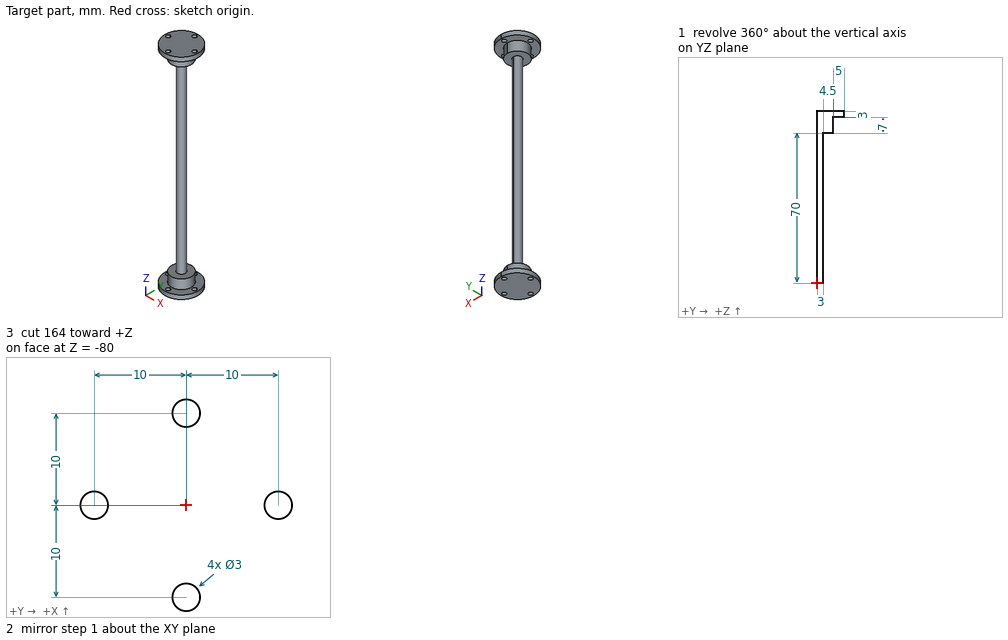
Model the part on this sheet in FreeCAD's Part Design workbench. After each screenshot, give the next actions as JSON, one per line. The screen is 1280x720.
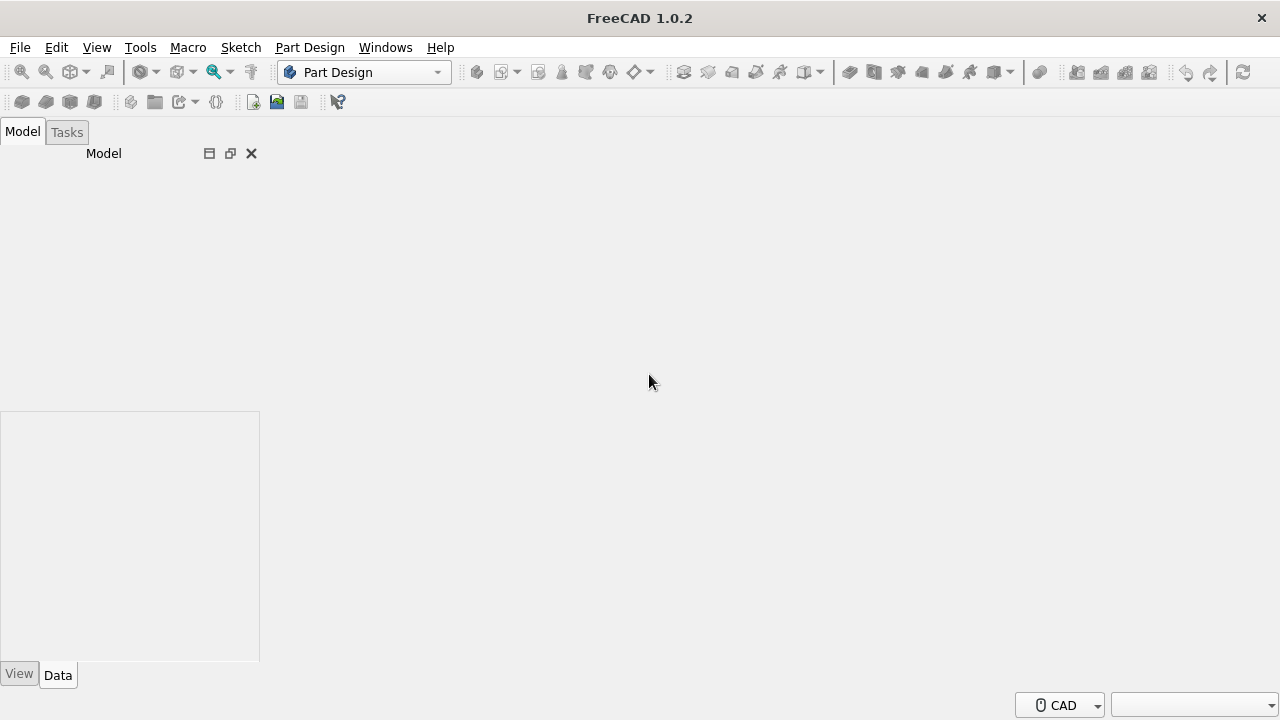
{"action": "left_click", "coordinate": [254, 102]}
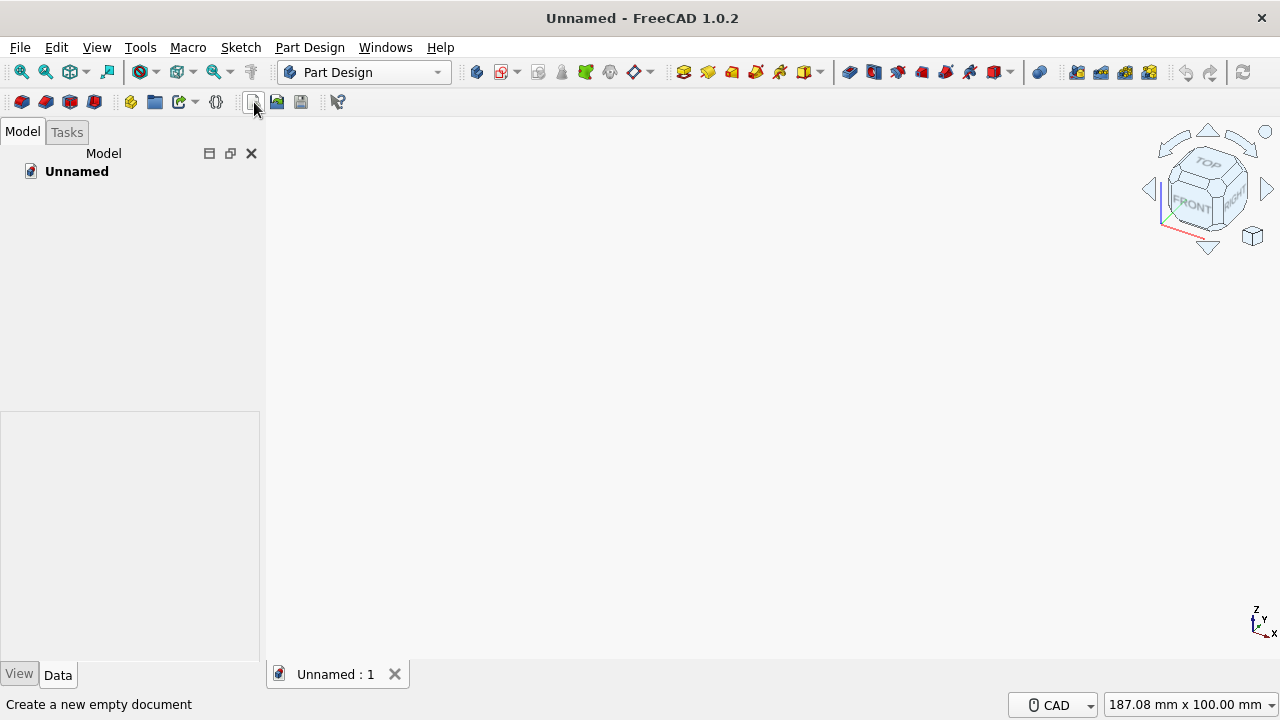
{"action": "left_click", "coordinate": [502, 72]}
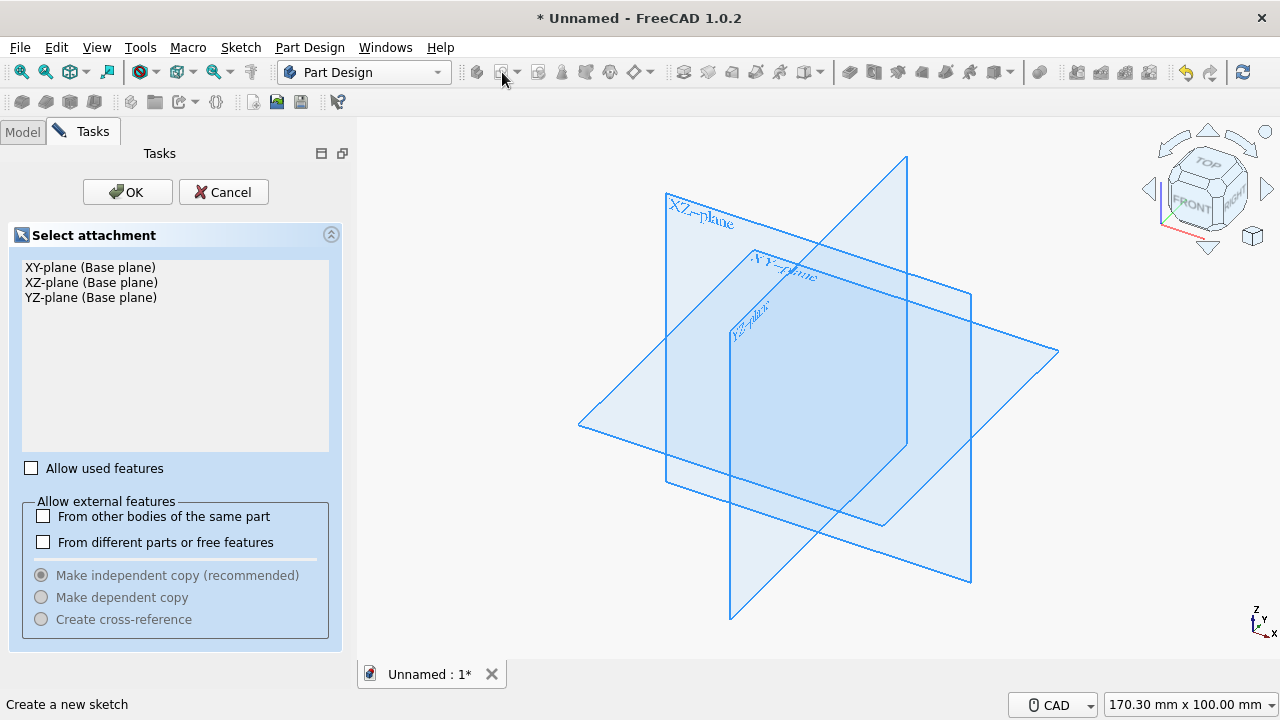
{"action": "left_click", "coordinate": [82, 298]}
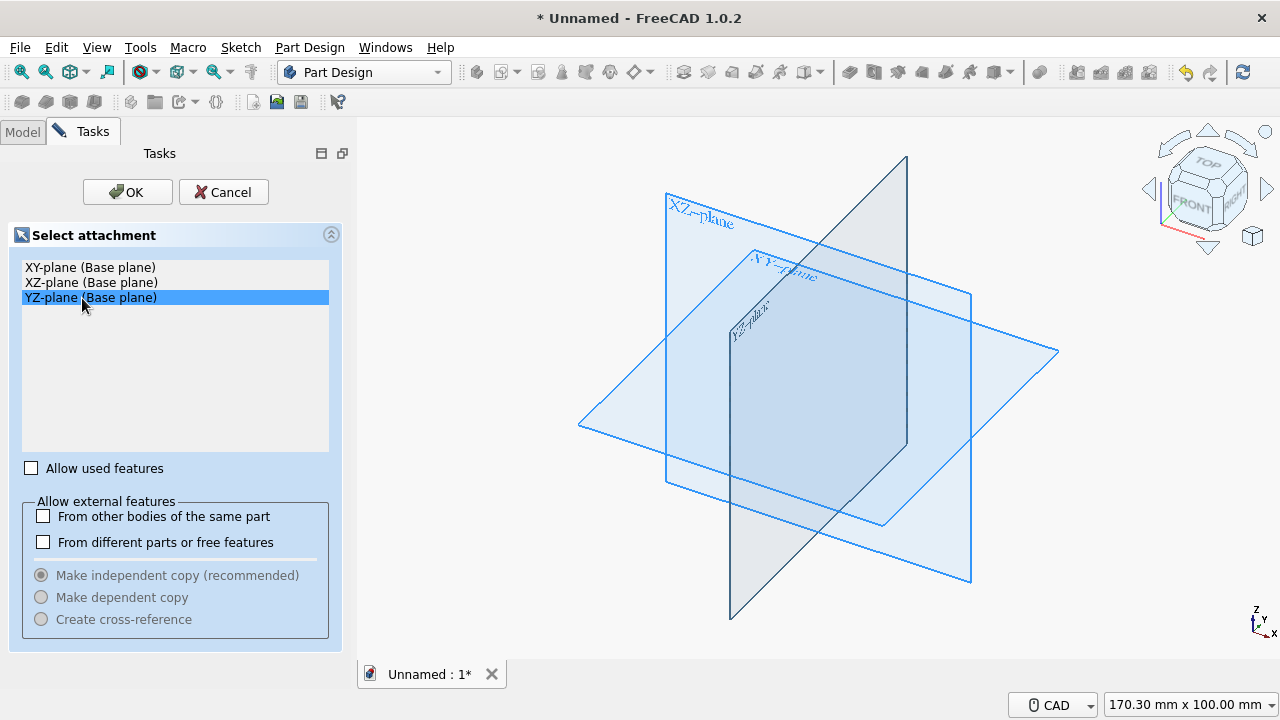
{"action": "left_click", "coordinate": [128, 192]}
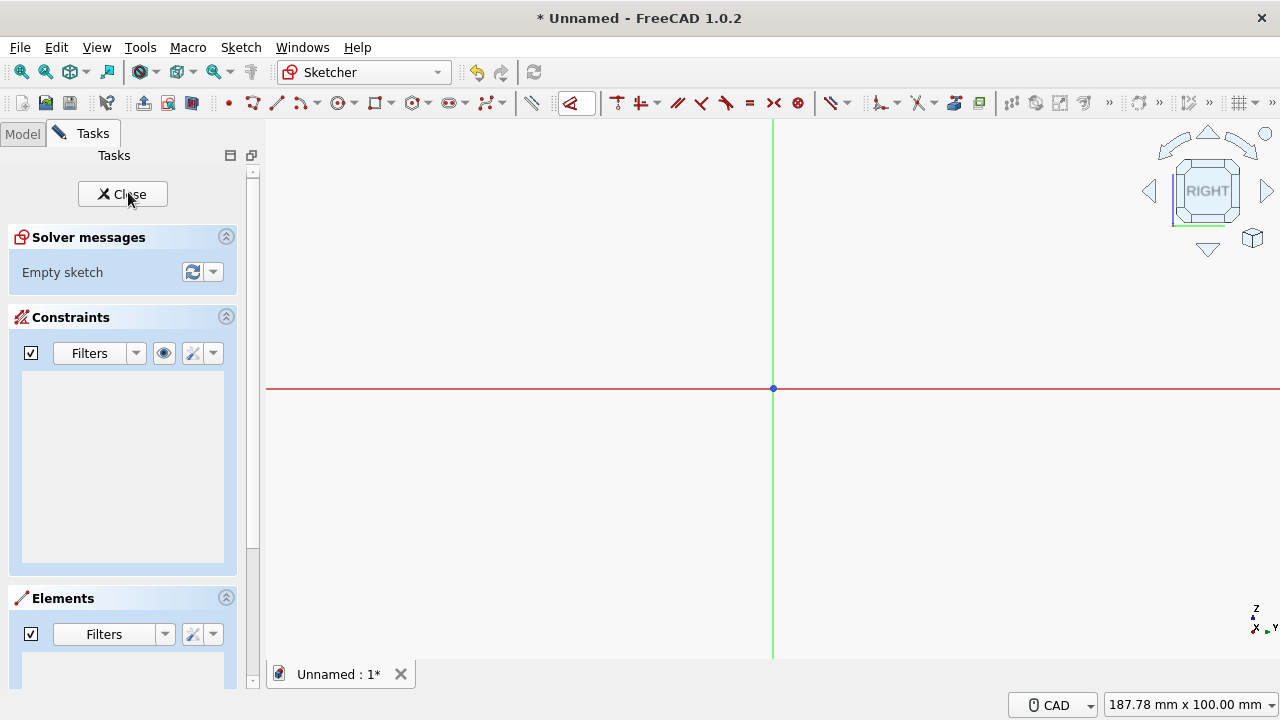
{"action": "scroll", "coordinate": [497, 631], "scroll_direction": "down", "scroll_amount": 2}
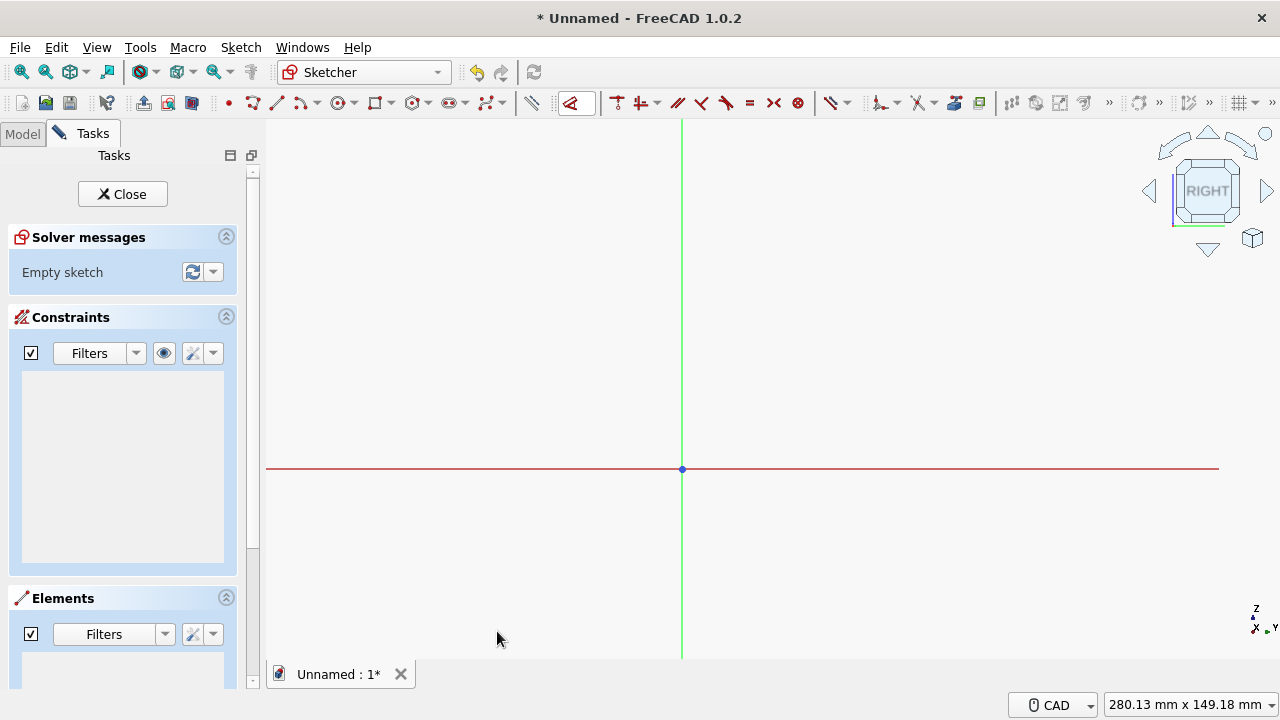
{"action": "left_click", "coordinate": [254, 104]}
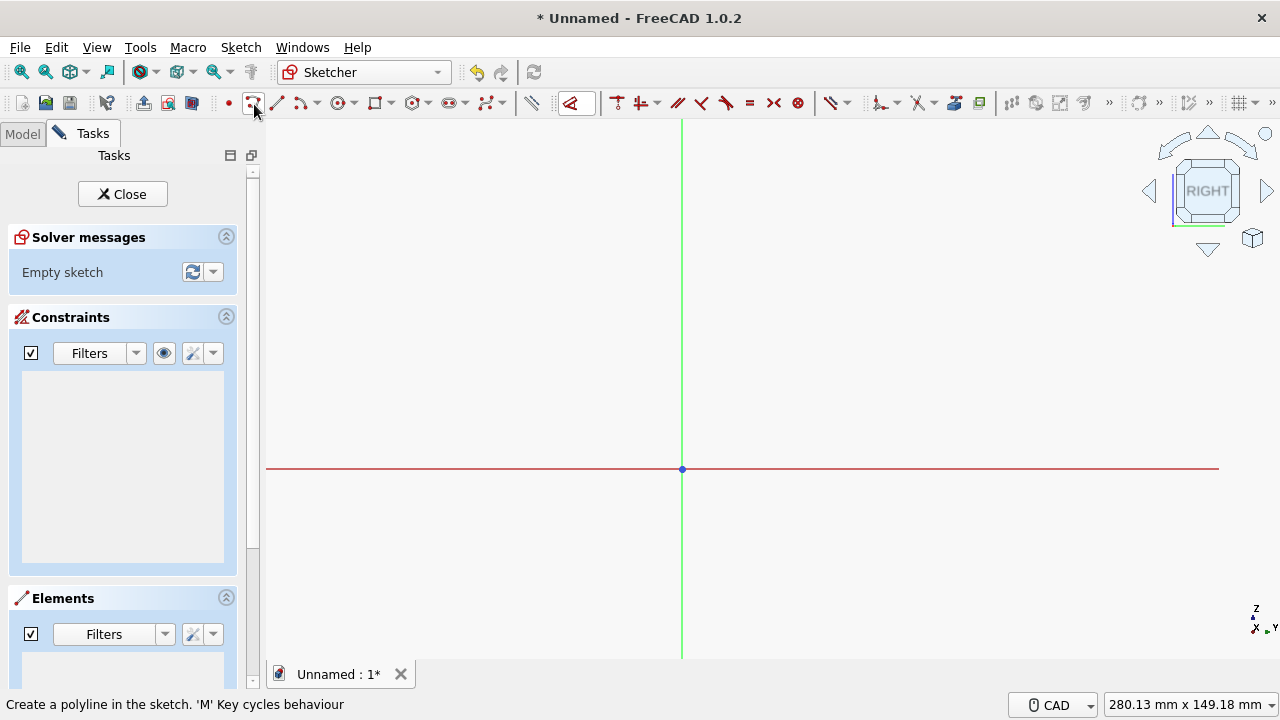
{"action": "left_click", "coordinate": [682, 469]}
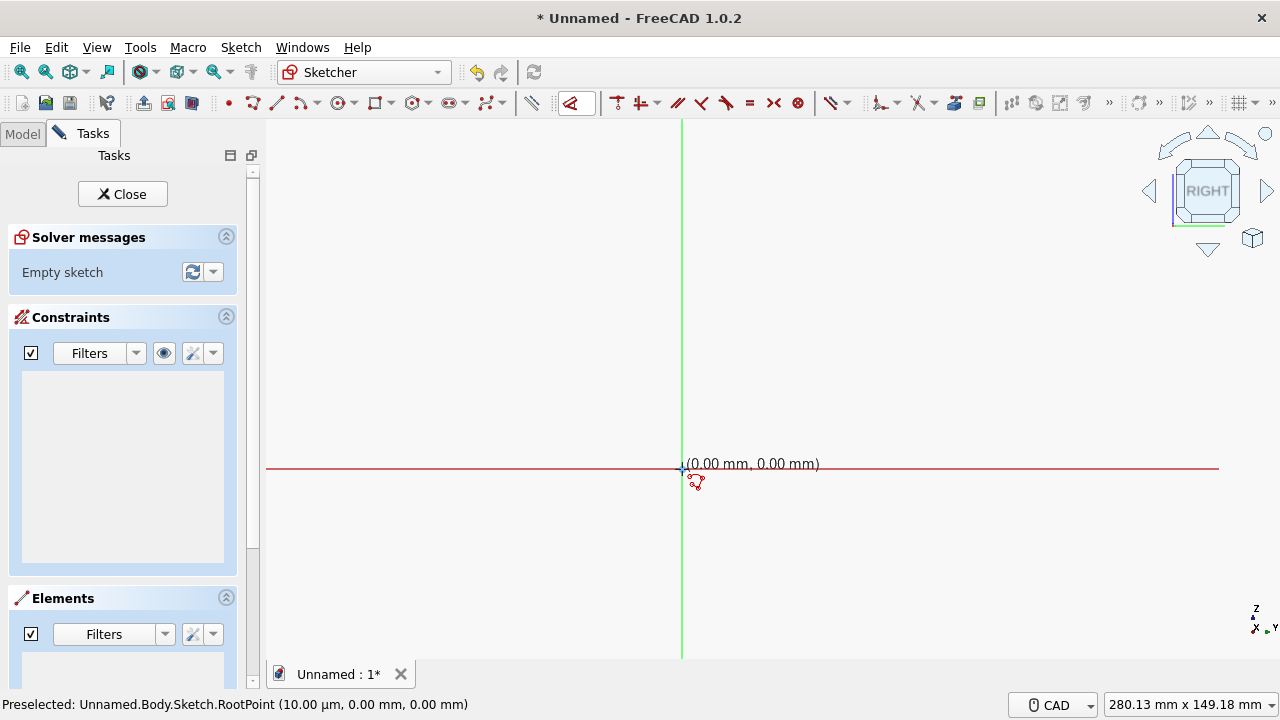
{"action": "scroll", "coordinate": [693, 469], "scroll_direction": "up", "scroll_amount": 2}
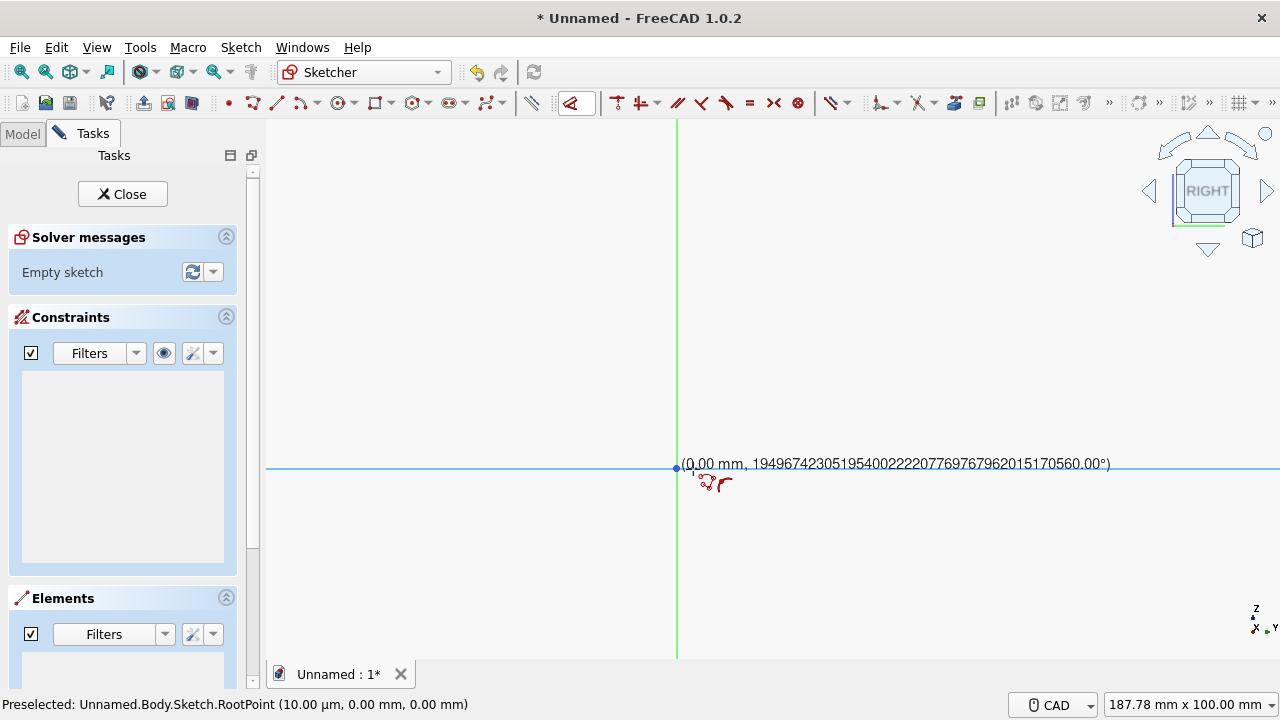
{"action": "left_click", "coordinate": [693, 460]}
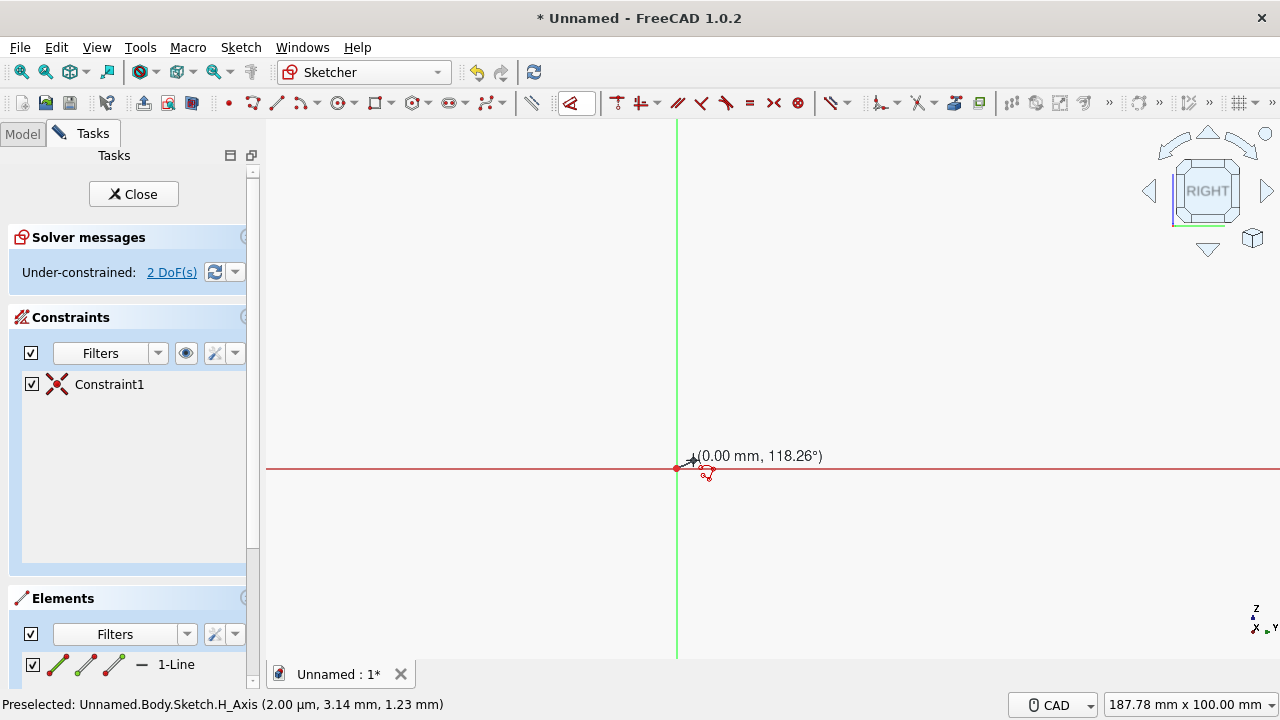
{"action": "scroll", "coordinate": [693, 631], "scroll_direction": "down", "scroll_amount": 2}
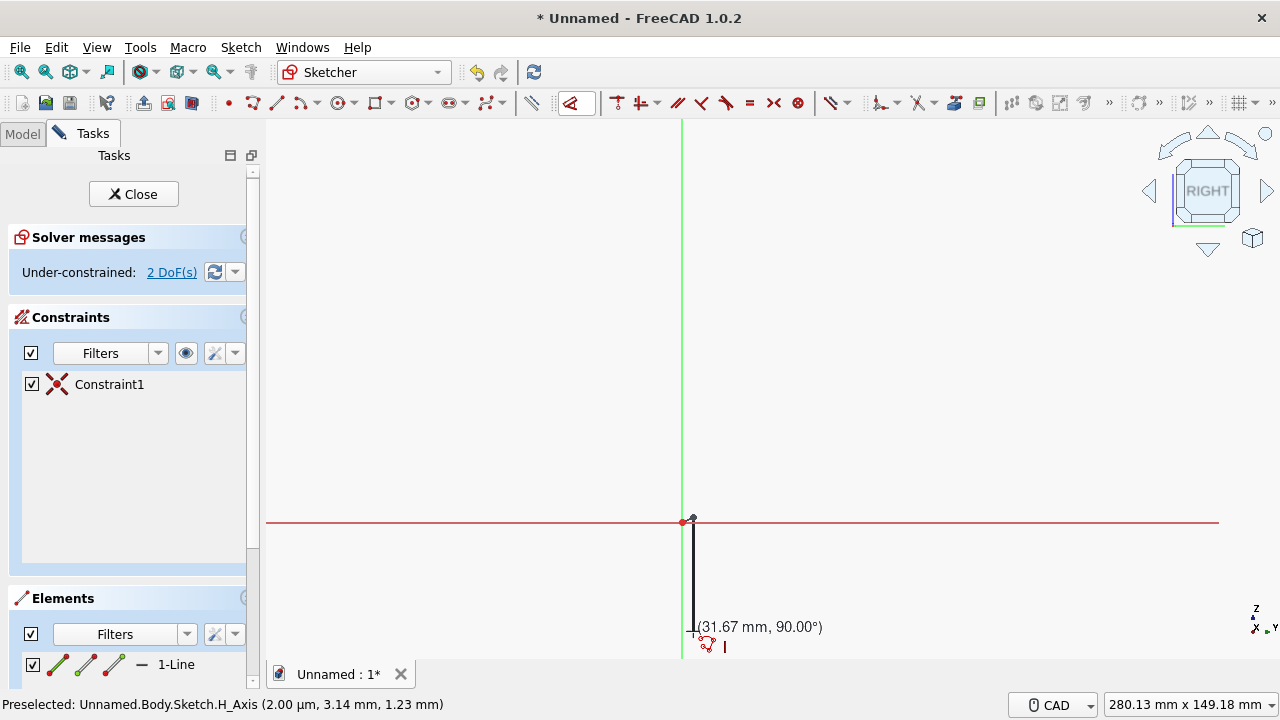
{"action": "scroll", "coordinate": [693, 269], "scroll_direction": "up", "scroll_amount": 2}